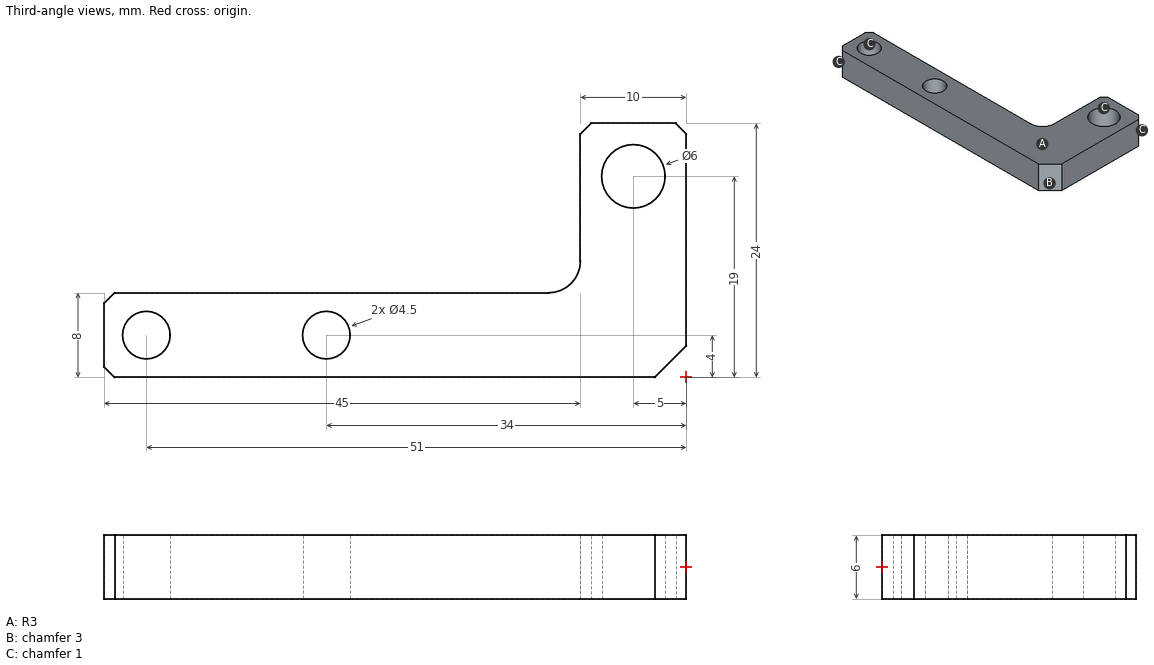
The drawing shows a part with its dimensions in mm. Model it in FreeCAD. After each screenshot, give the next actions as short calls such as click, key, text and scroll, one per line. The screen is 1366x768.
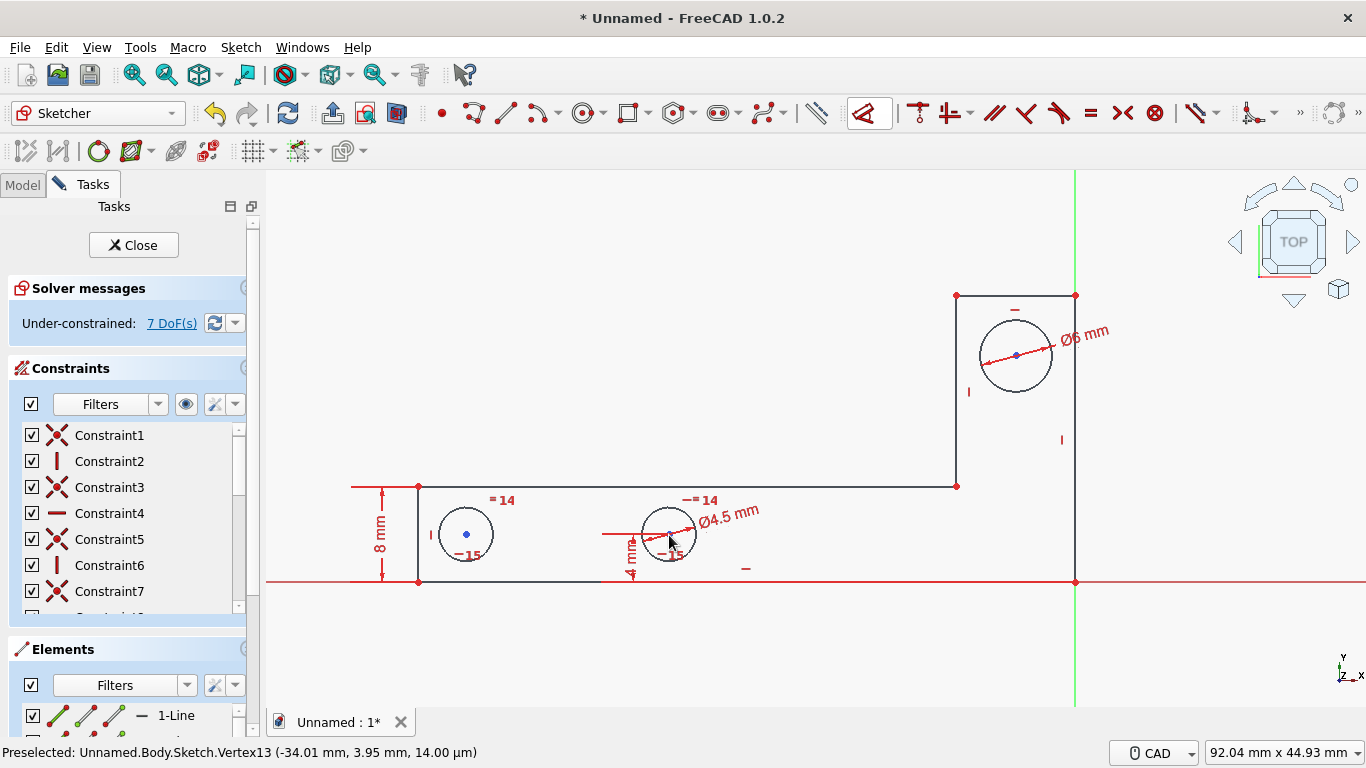
click(1016, 356)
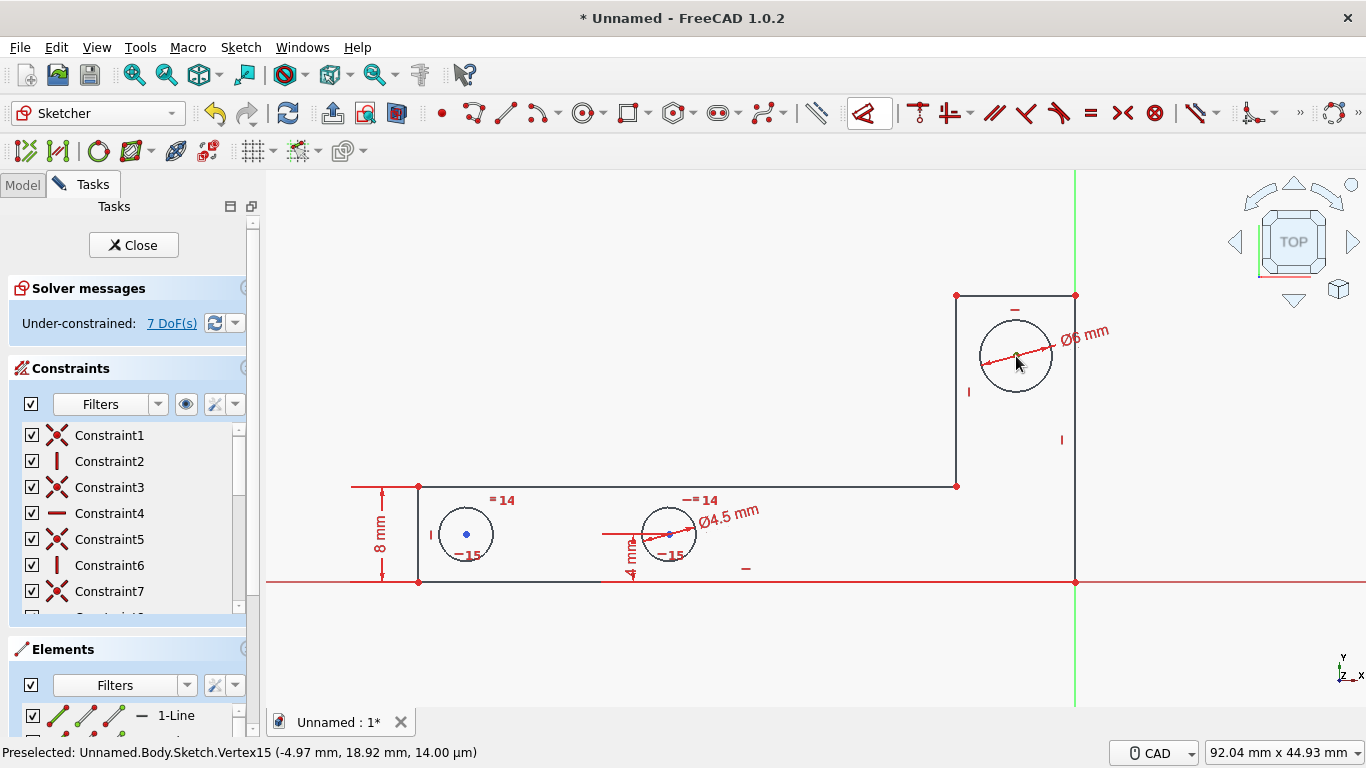
click(886, 114)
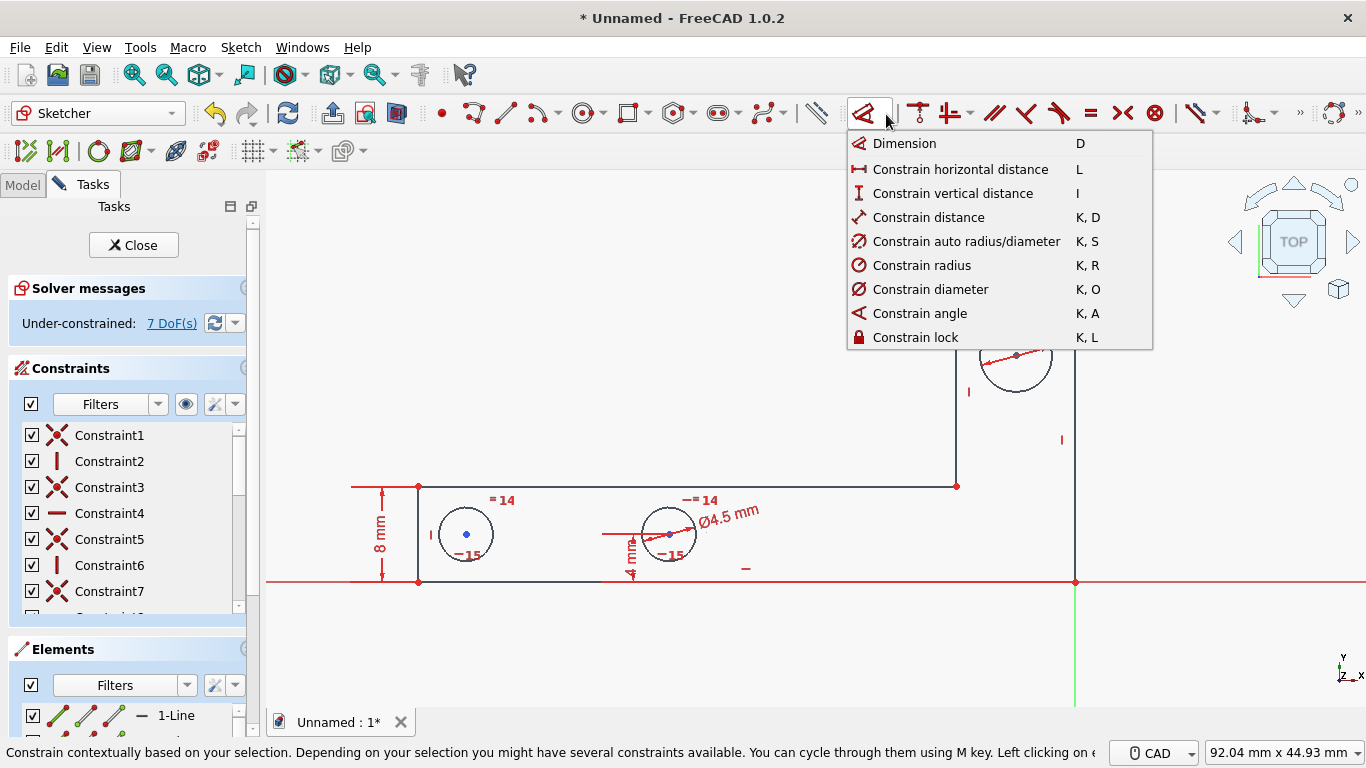
click(1000, 169)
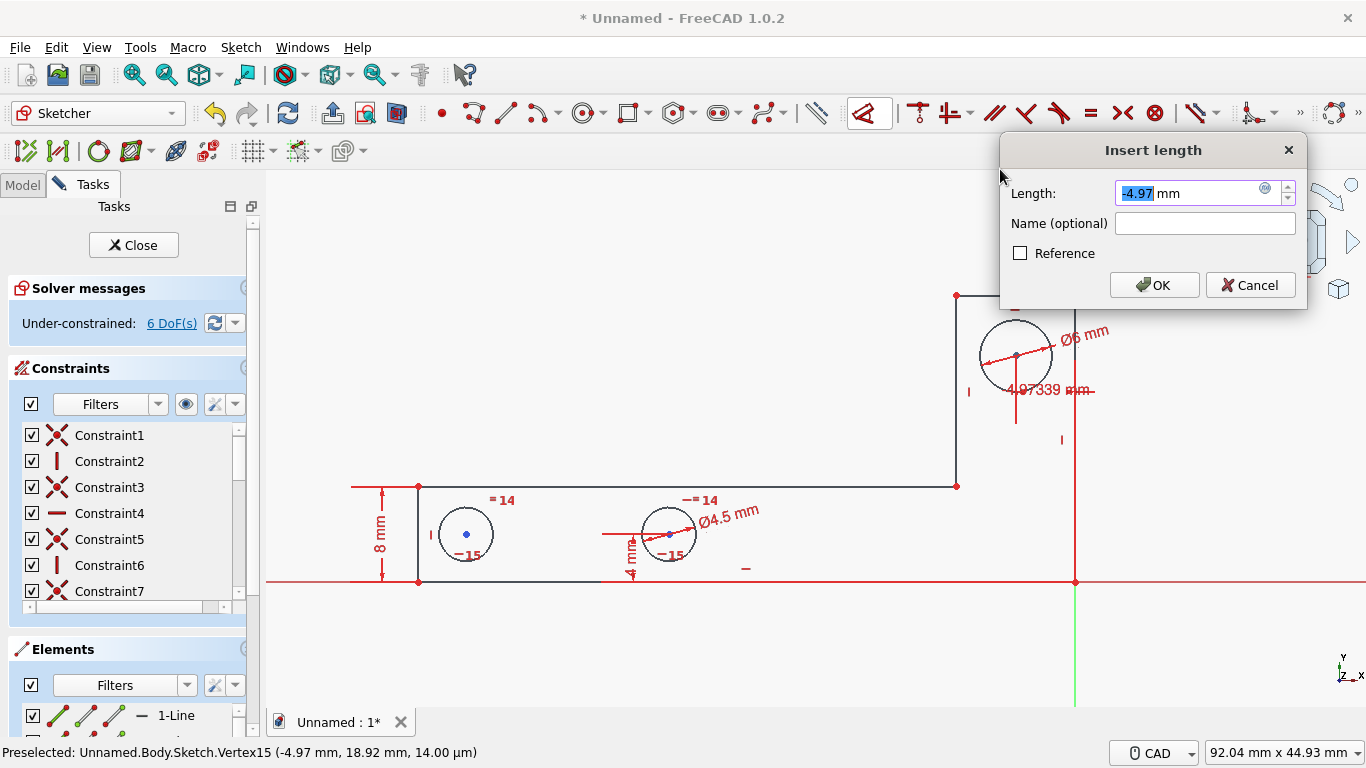
text(-5)
key(Return)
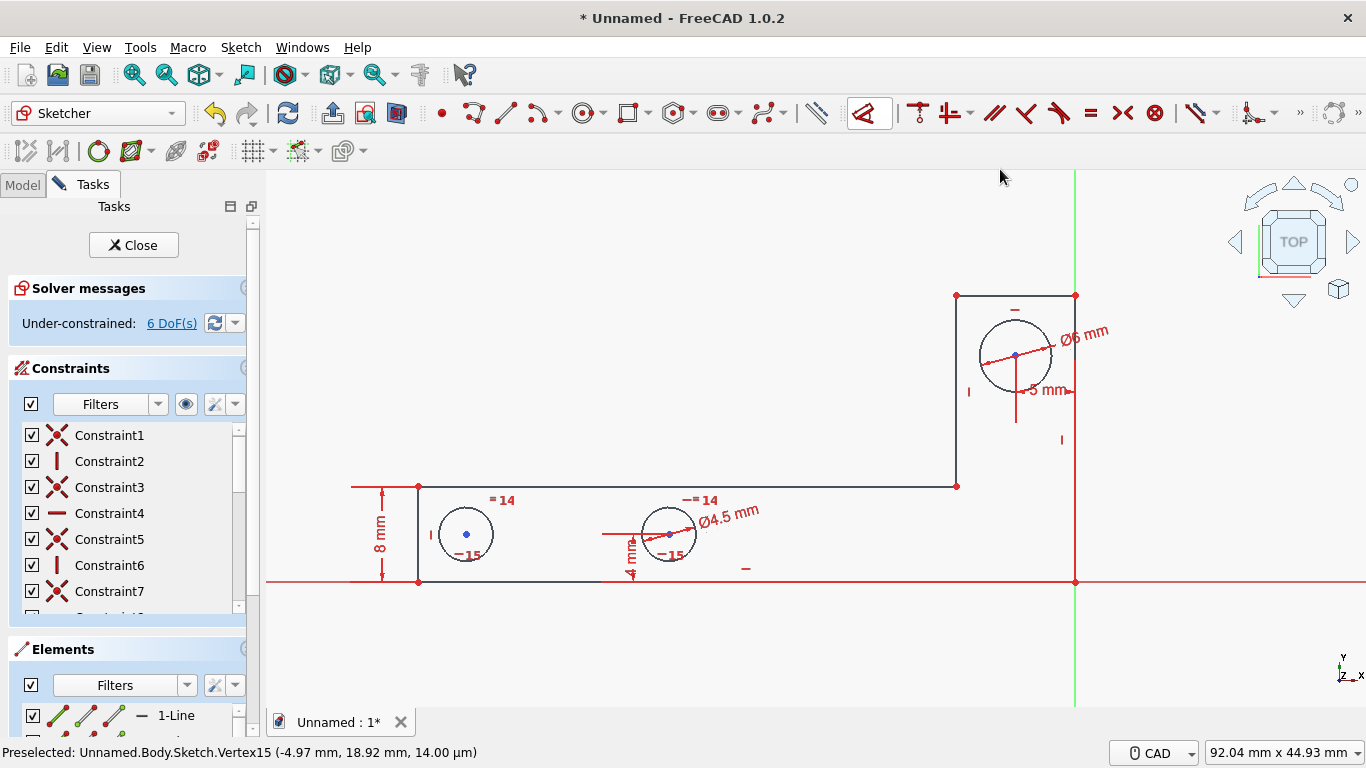
click(1075, 496)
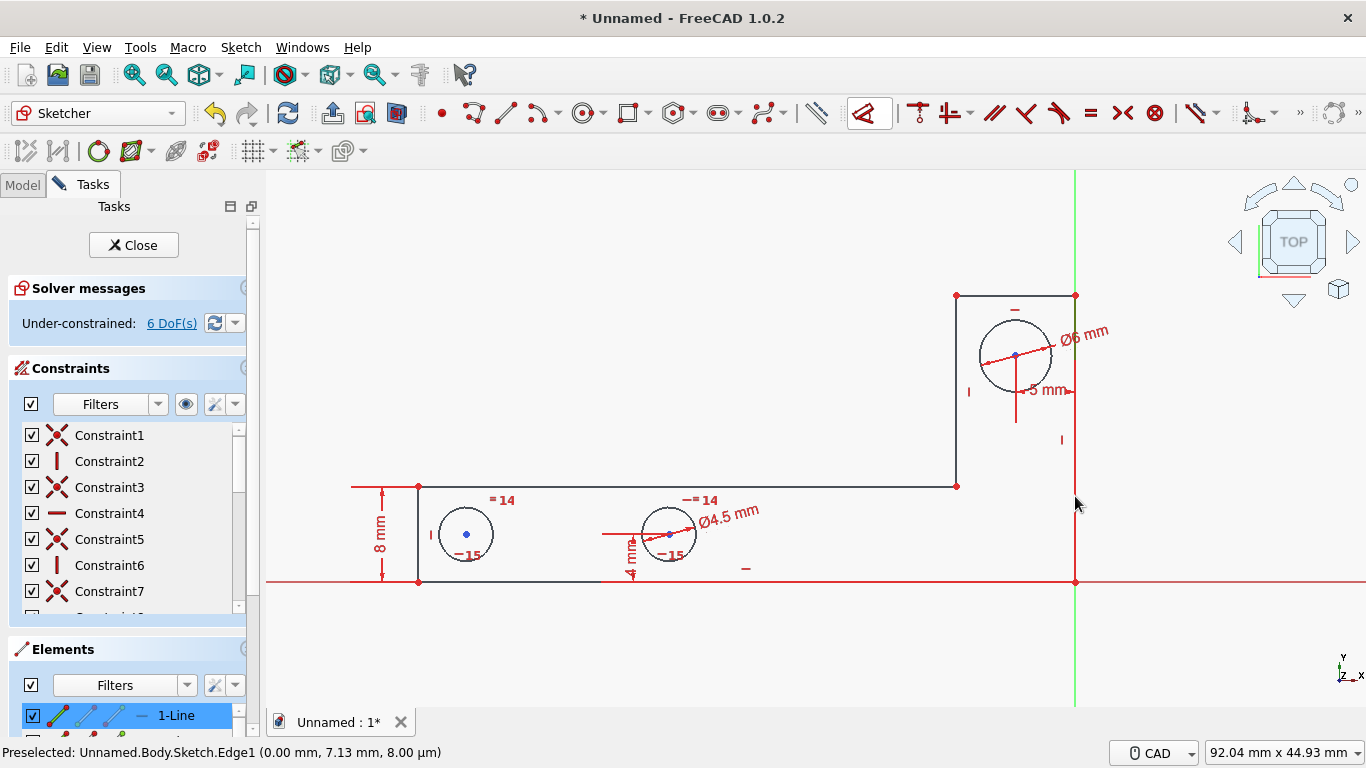
click(886, 114)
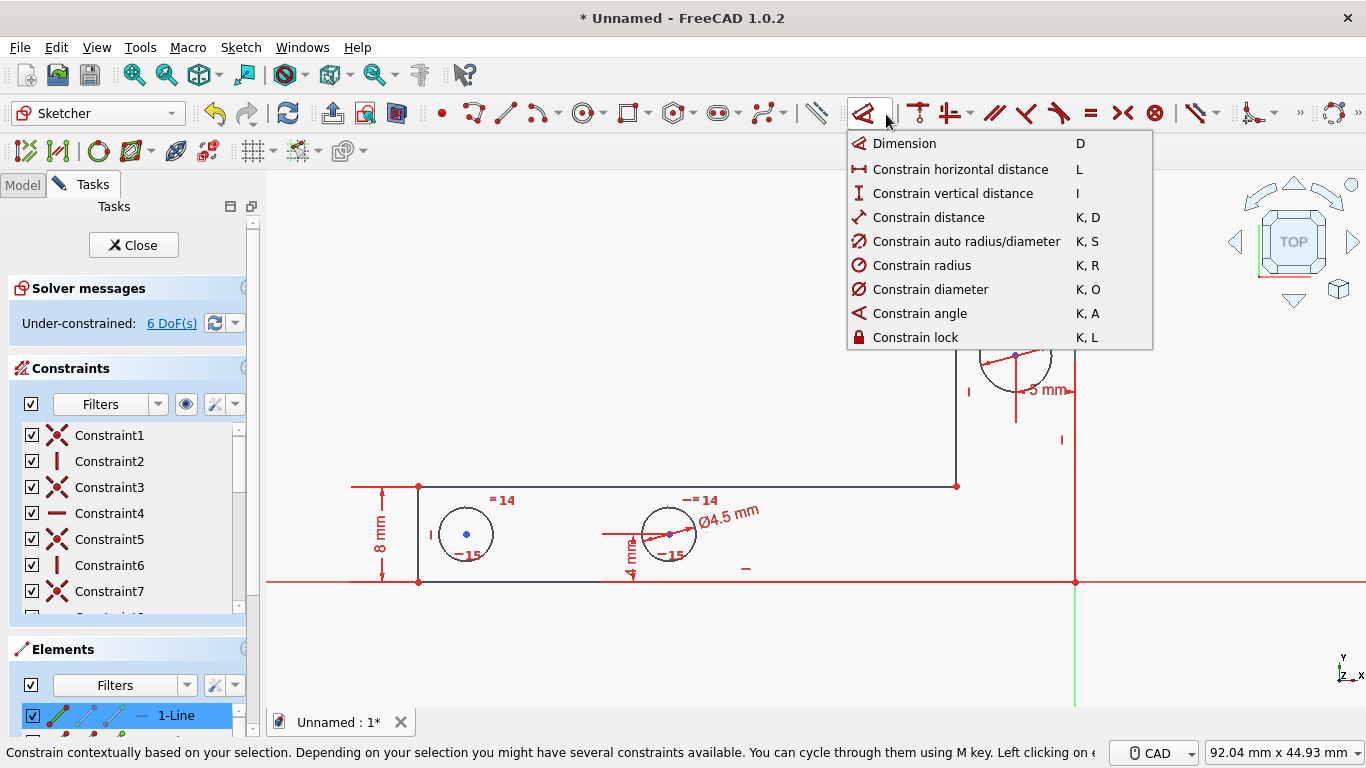
click(1000, 193)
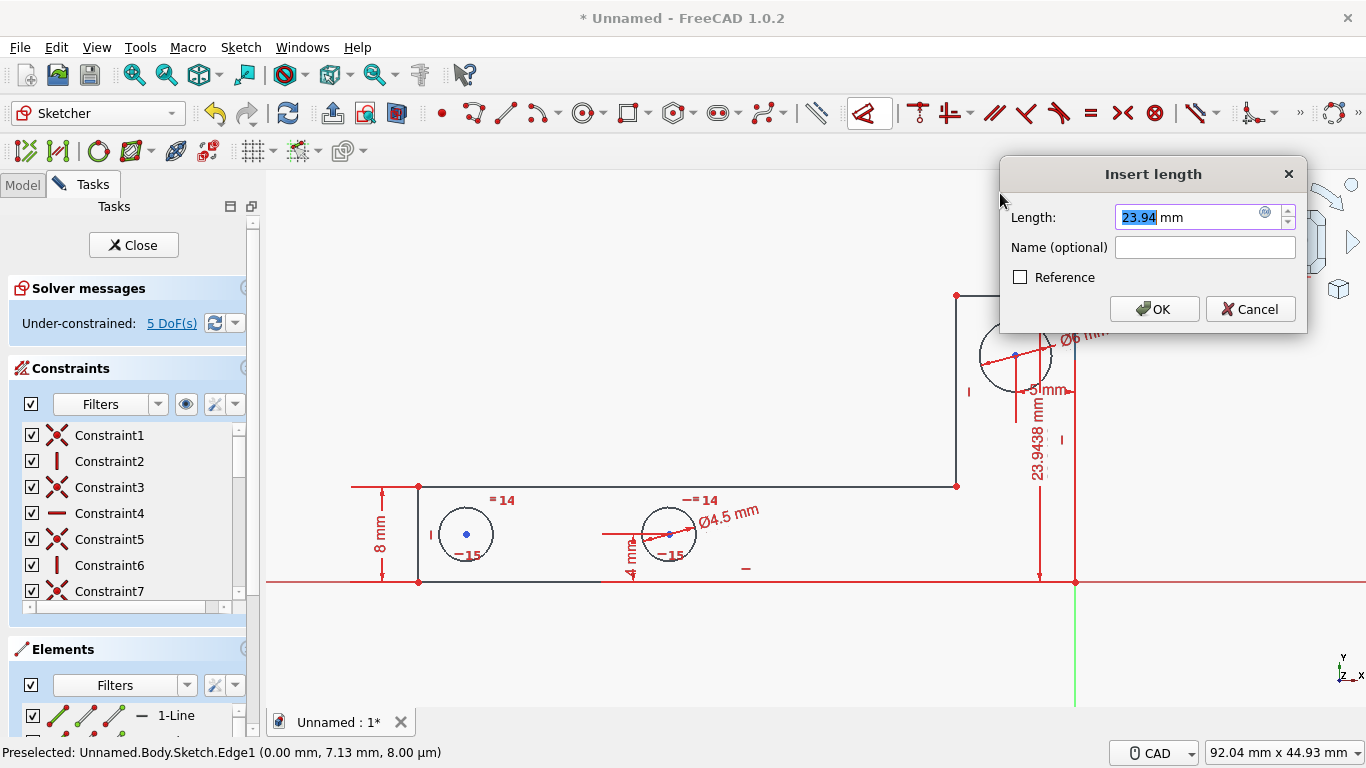
text(24)
key(Return)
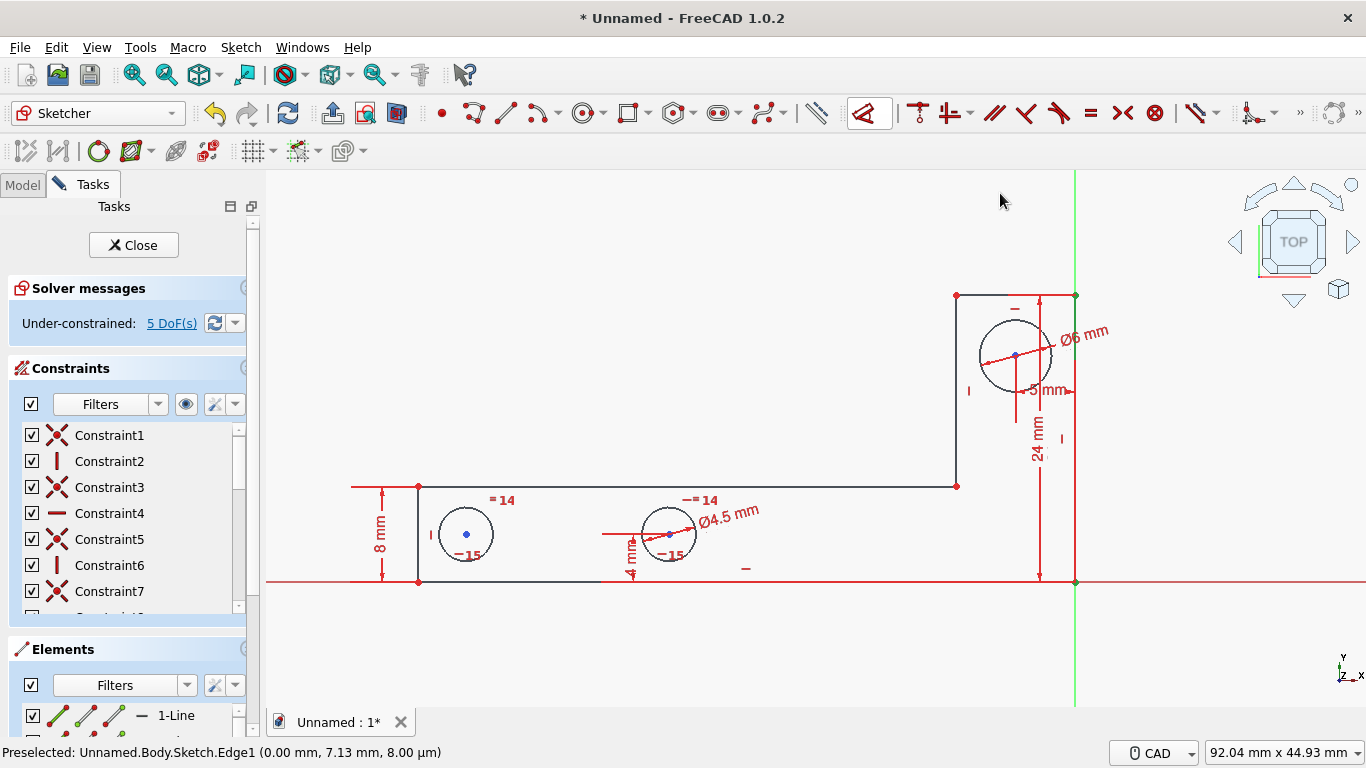
click(1040, 295)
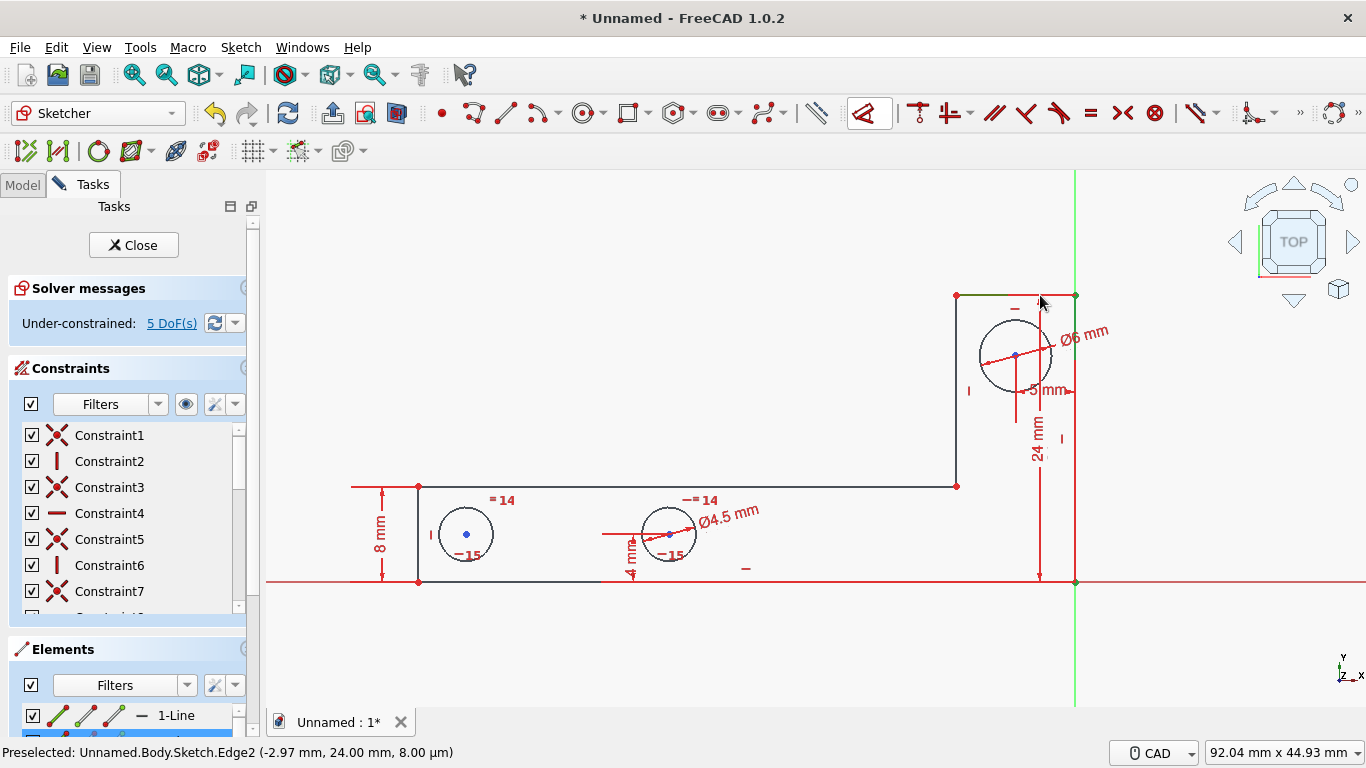
key(l)